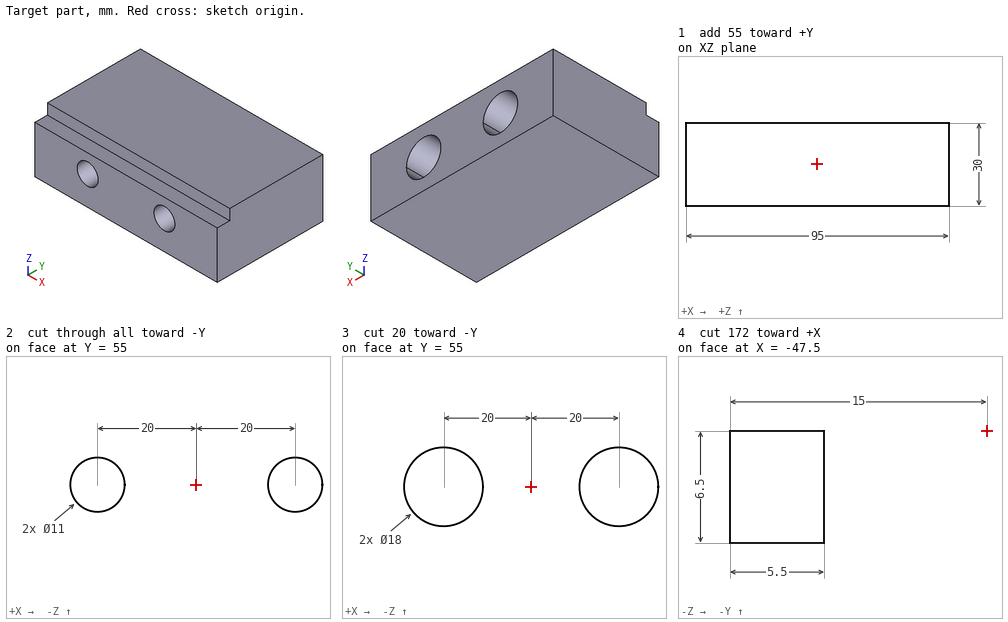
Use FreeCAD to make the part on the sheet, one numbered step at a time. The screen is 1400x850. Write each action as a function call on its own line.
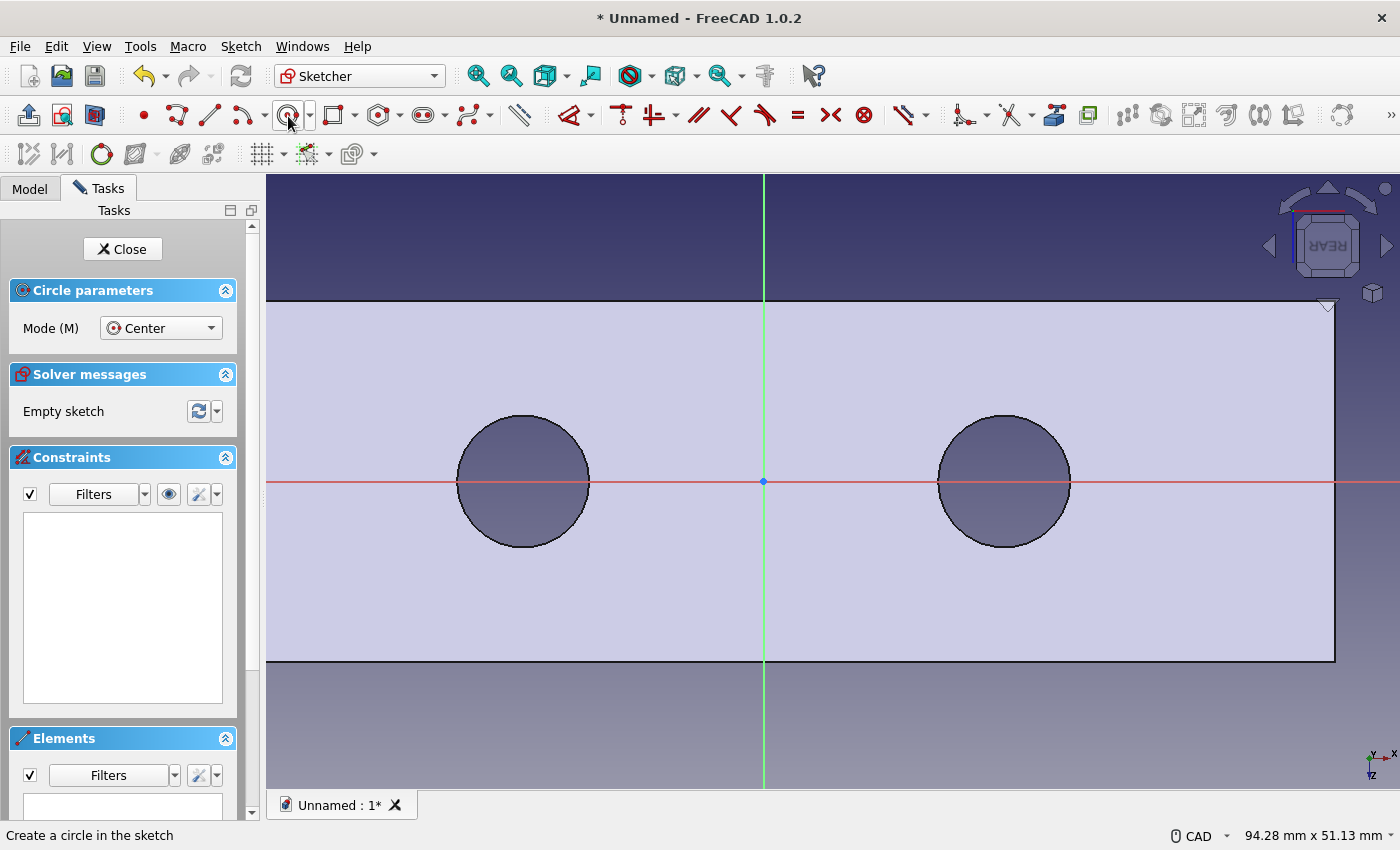
click(523, 481)
move(600, 405)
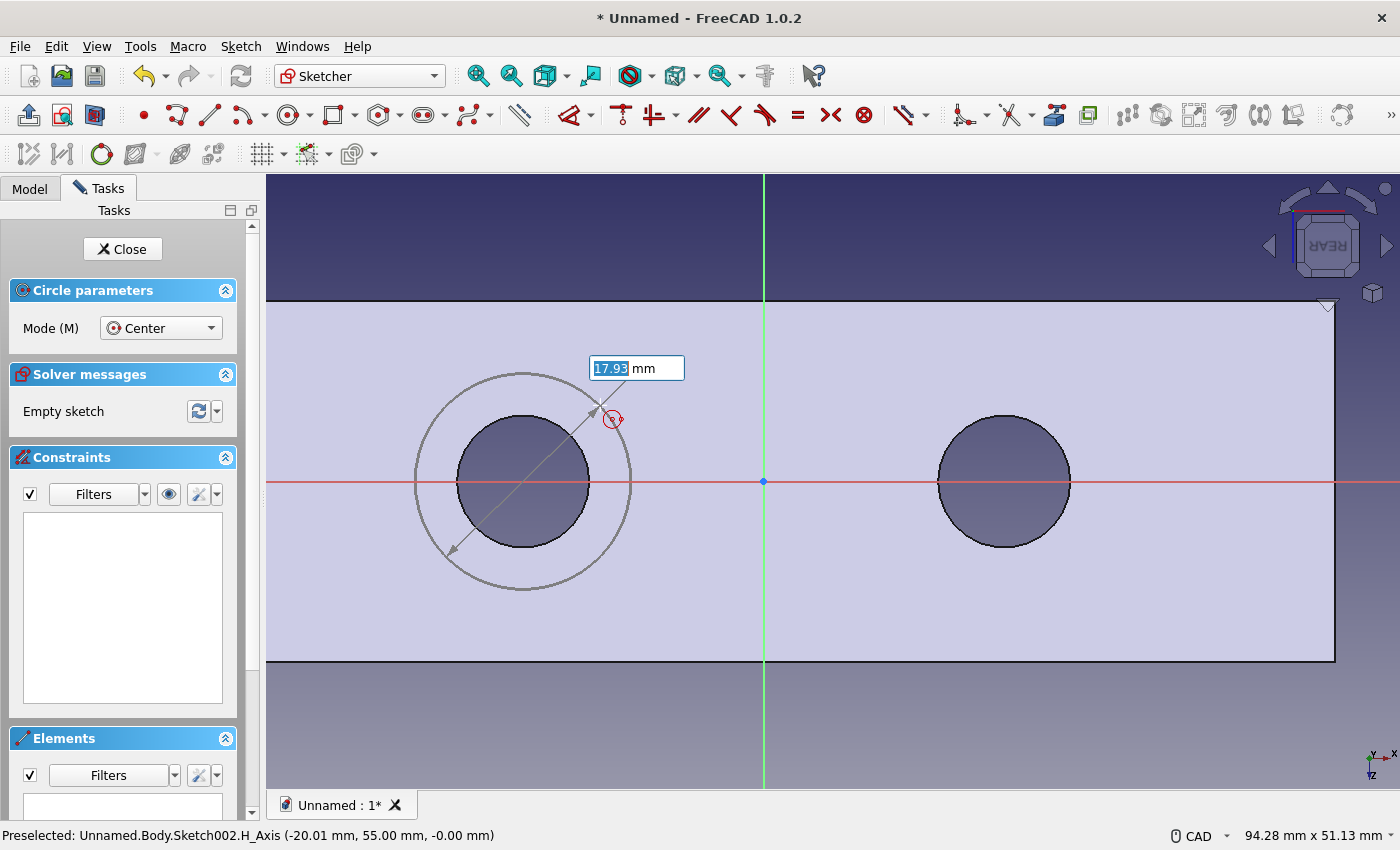
text(18)
key(Return)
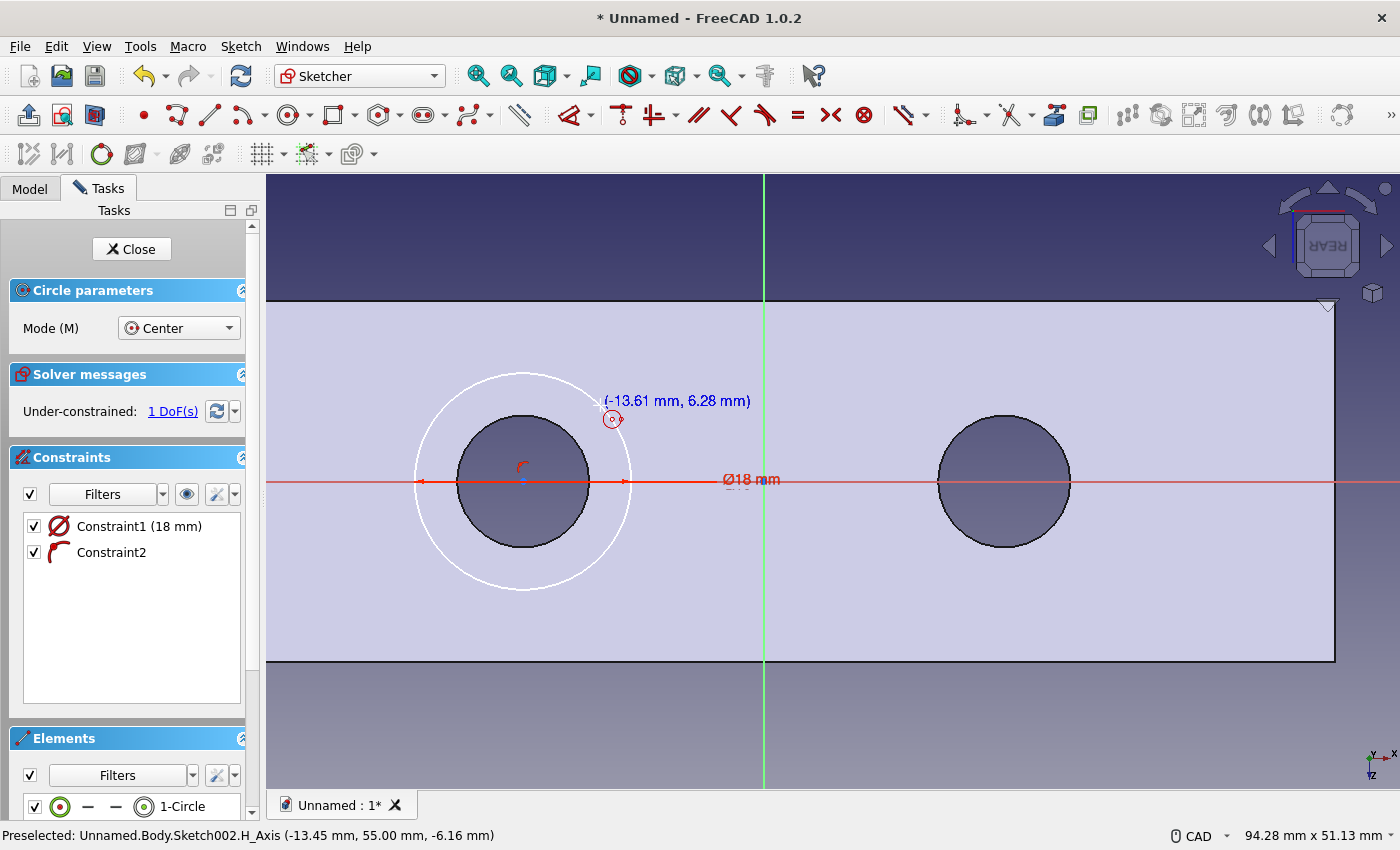
click(1004, 481)
move(1081, 405)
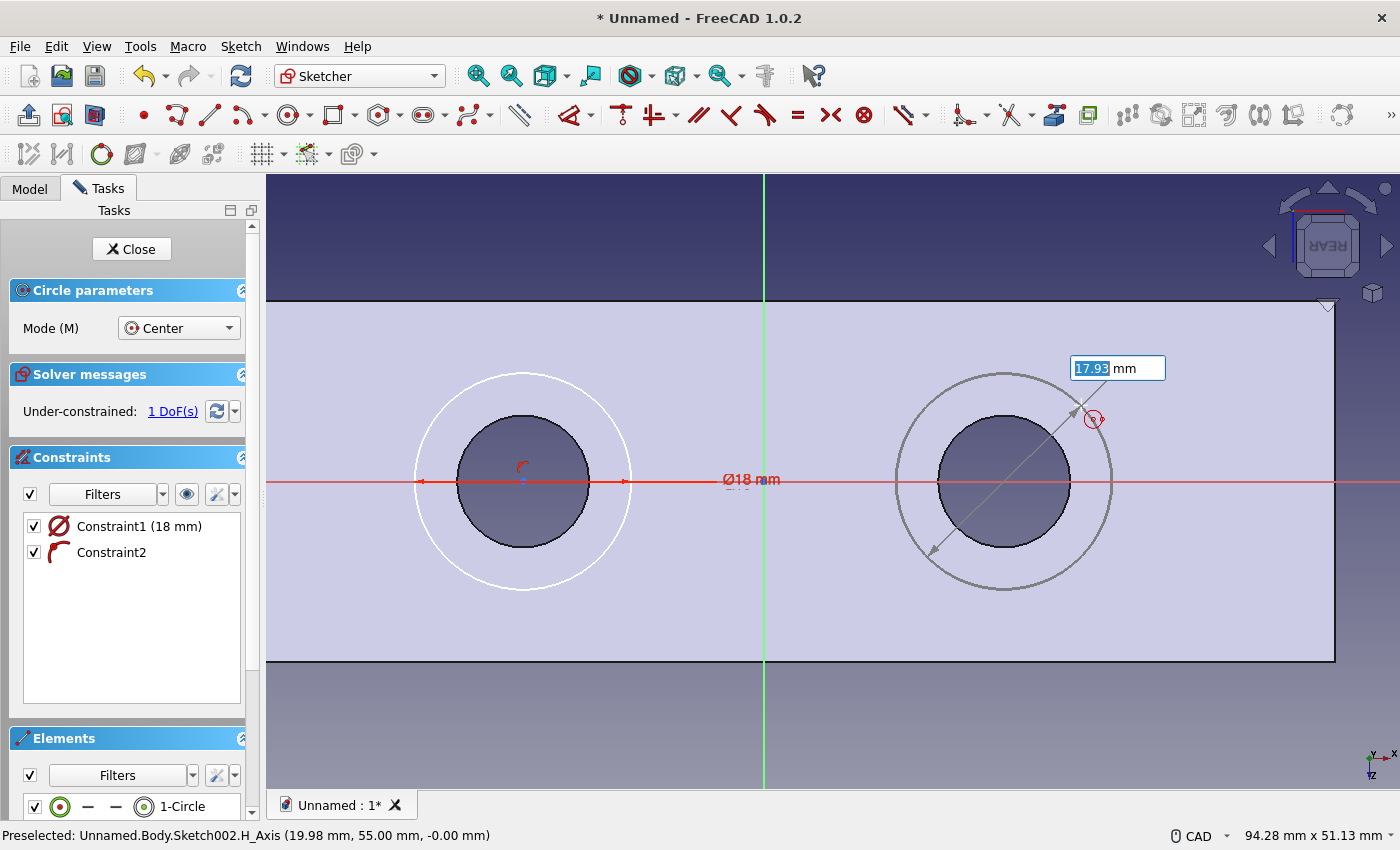
text(18)
key(Return)
key(Escape)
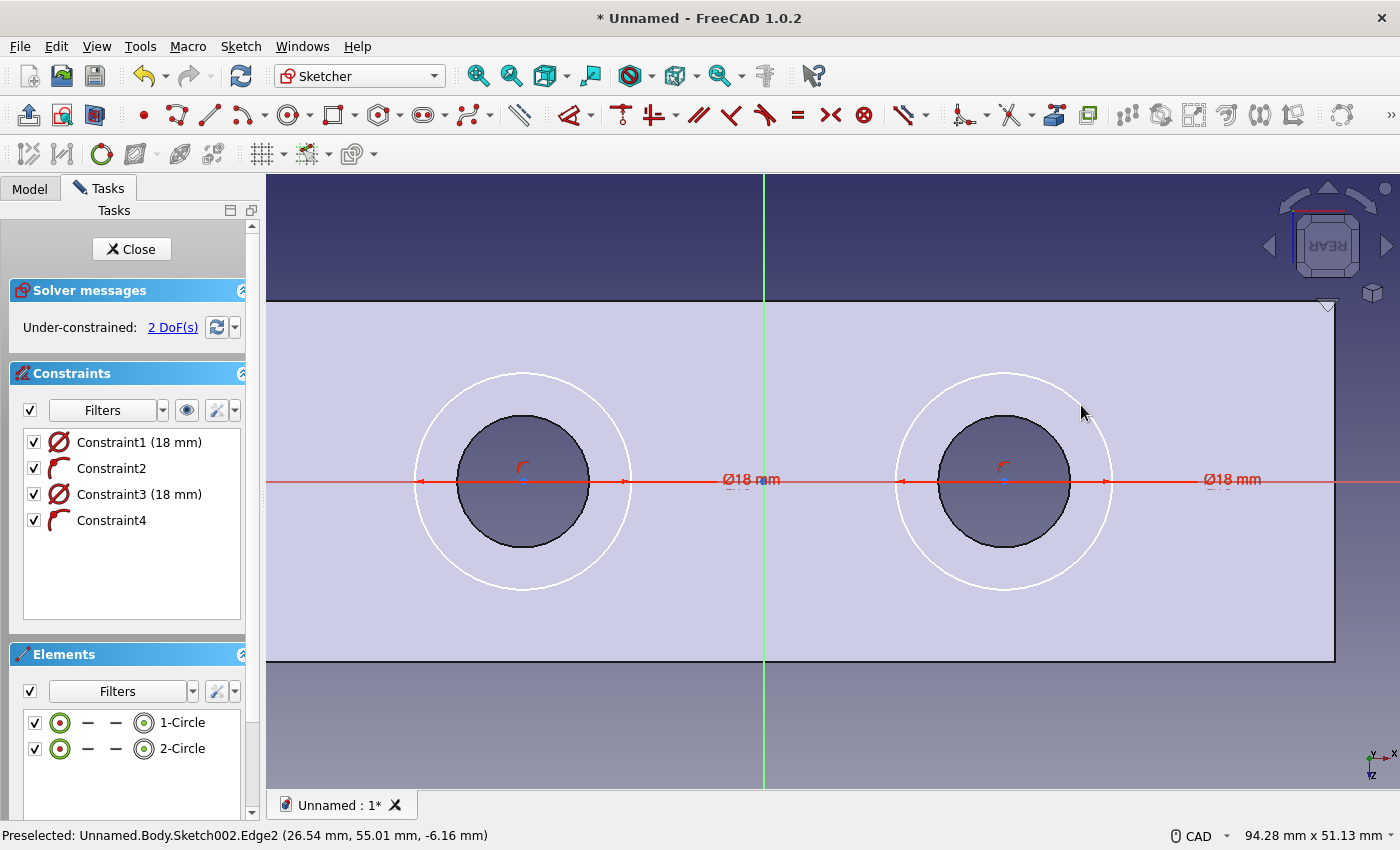
click(568, 116)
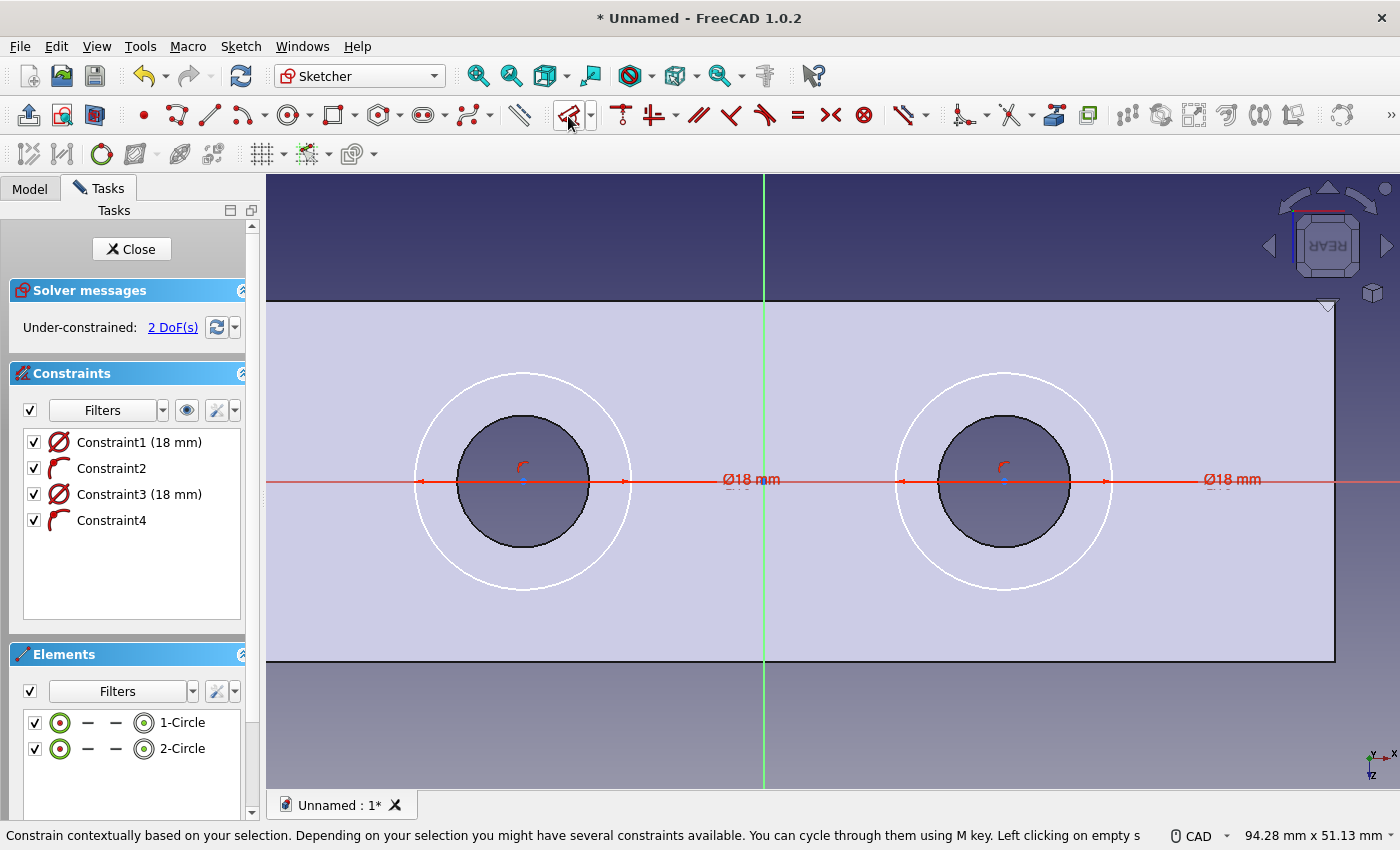
click(523, 481)
click(643, 515)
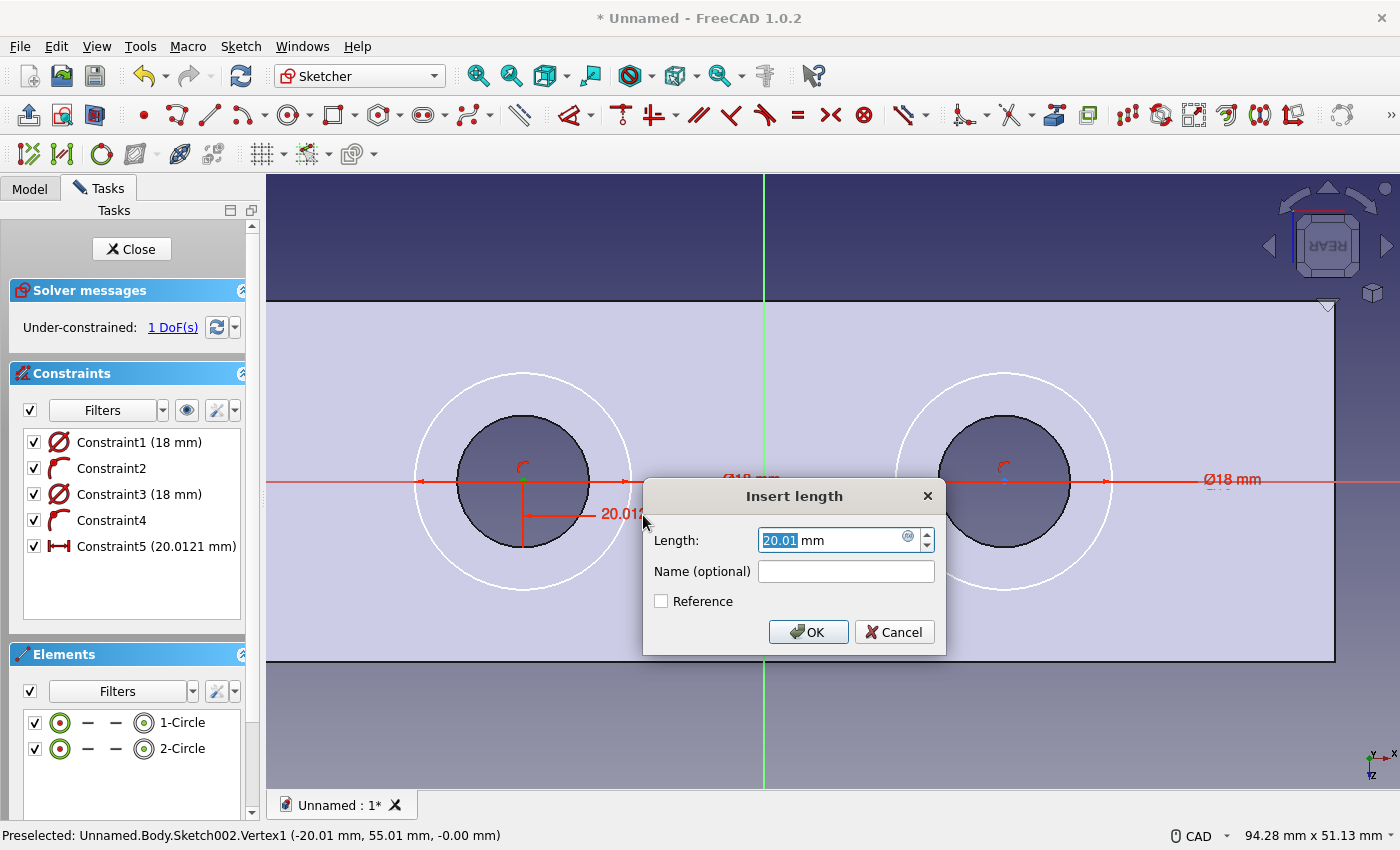
text(20)
key(Return)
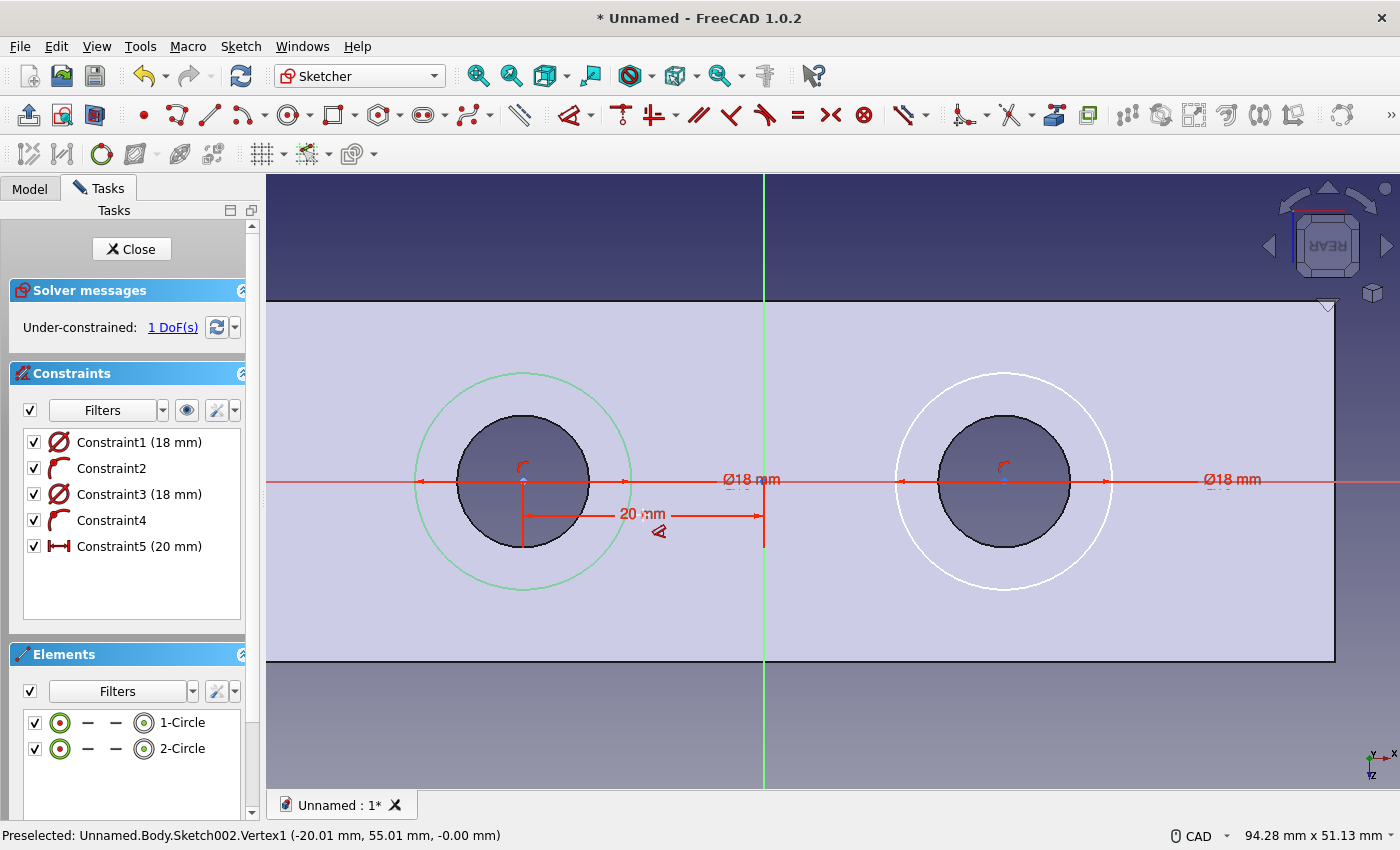
click(1004, 481)
click(884, 515)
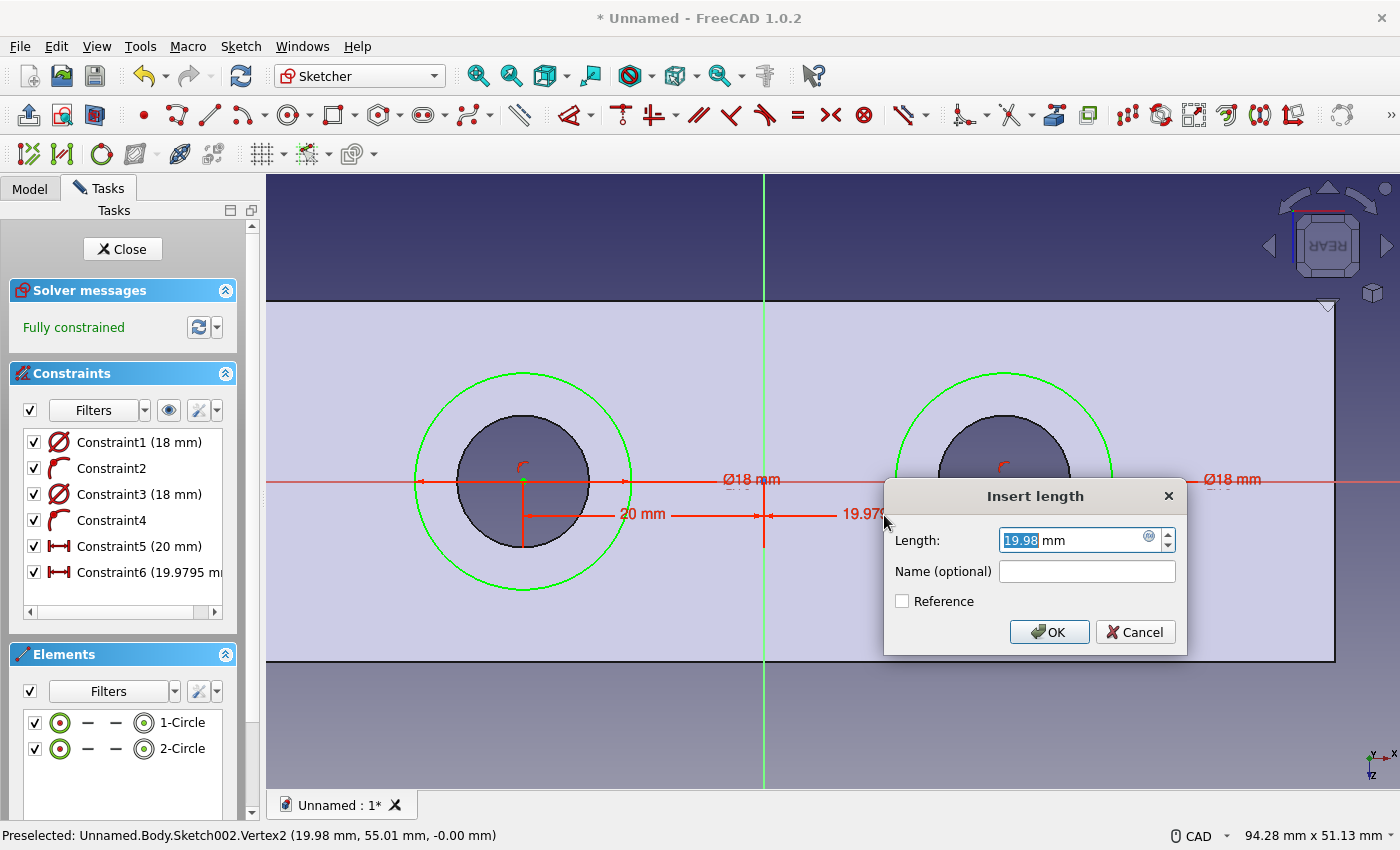
text(20)
key(Return)
key(Escape)